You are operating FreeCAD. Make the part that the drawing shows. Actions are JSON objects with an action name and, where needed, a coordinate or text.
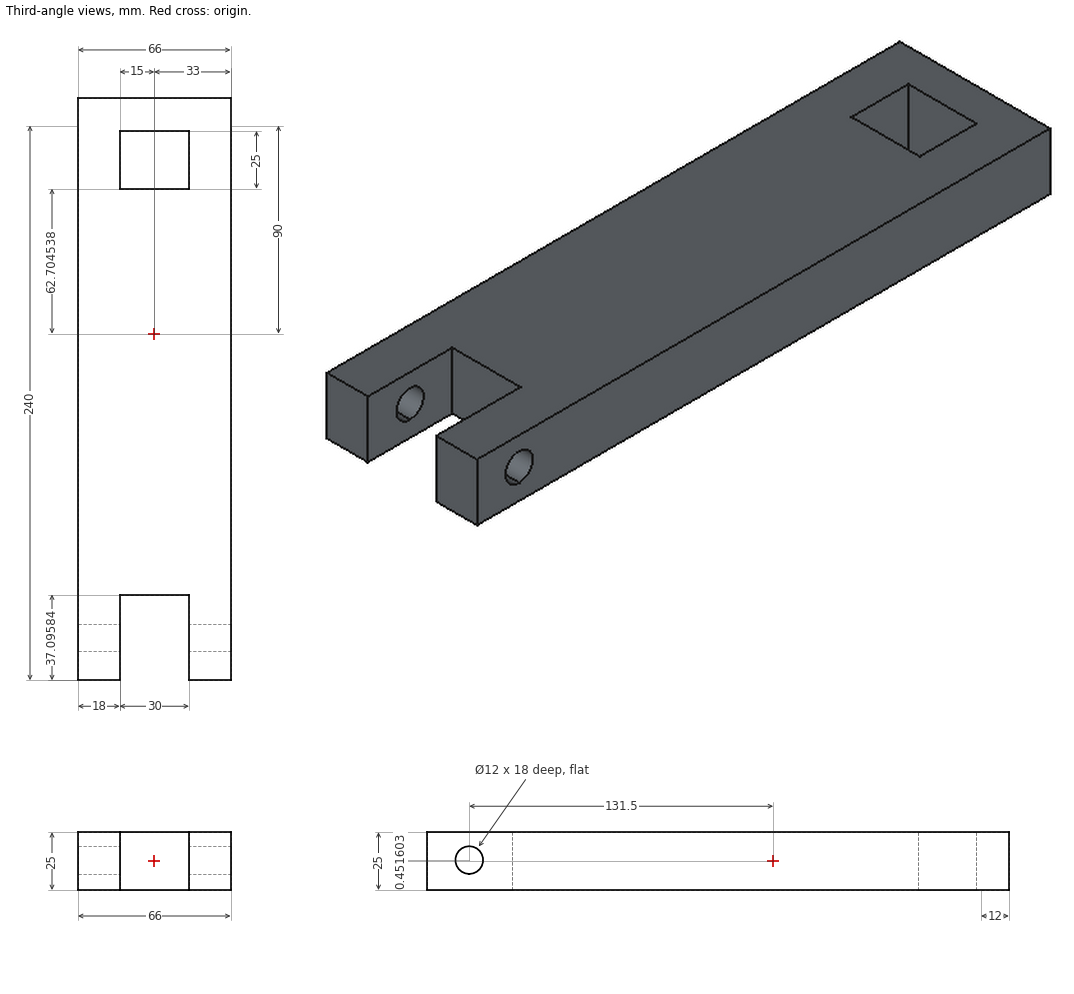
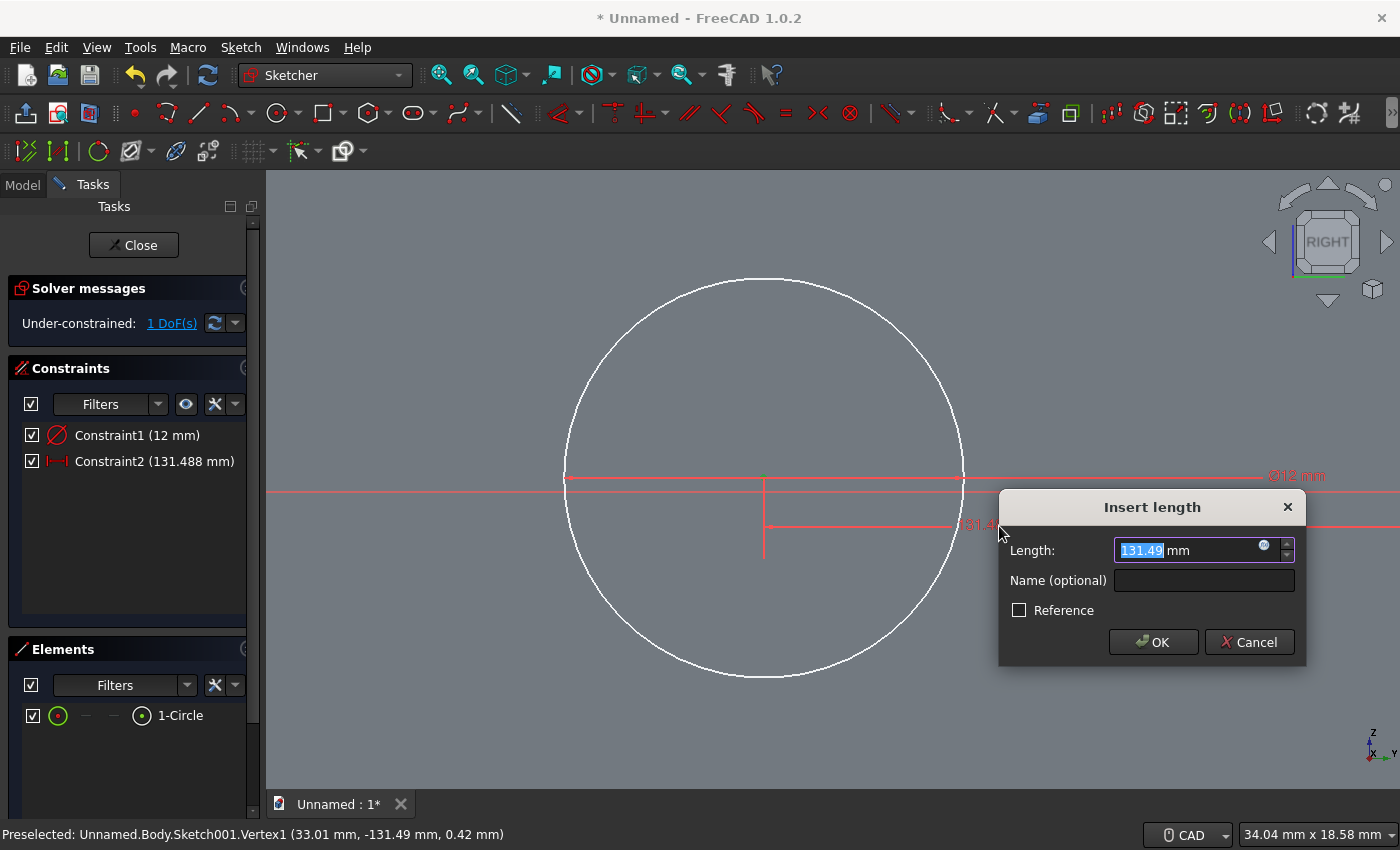
{"action": "type", "text": "131.5"}
{"action": "key", "text": "Return"}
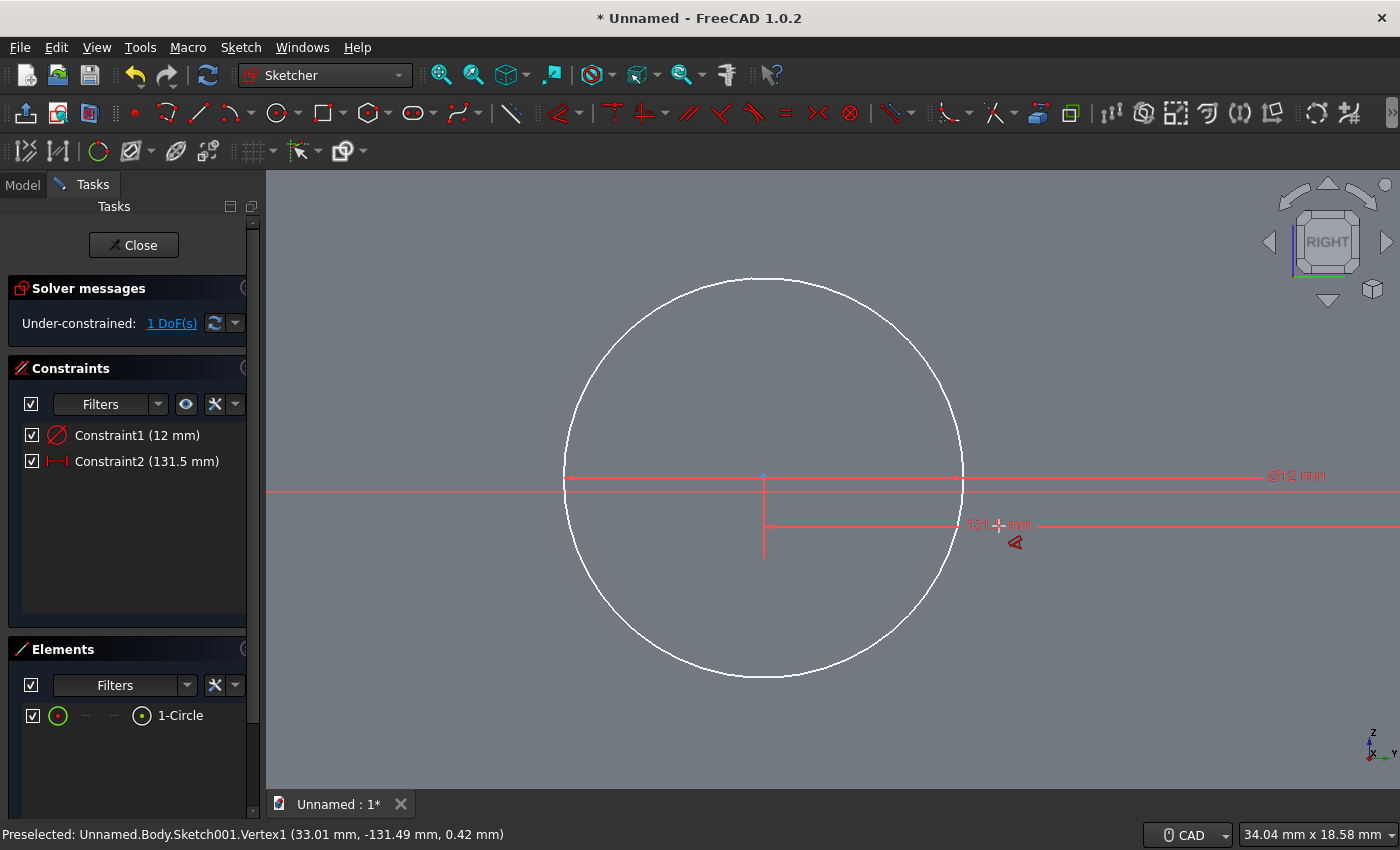
{"action": "scroll", "coordinate": [764, 478], "scroll_direction": "up", "scroll_amount": 5}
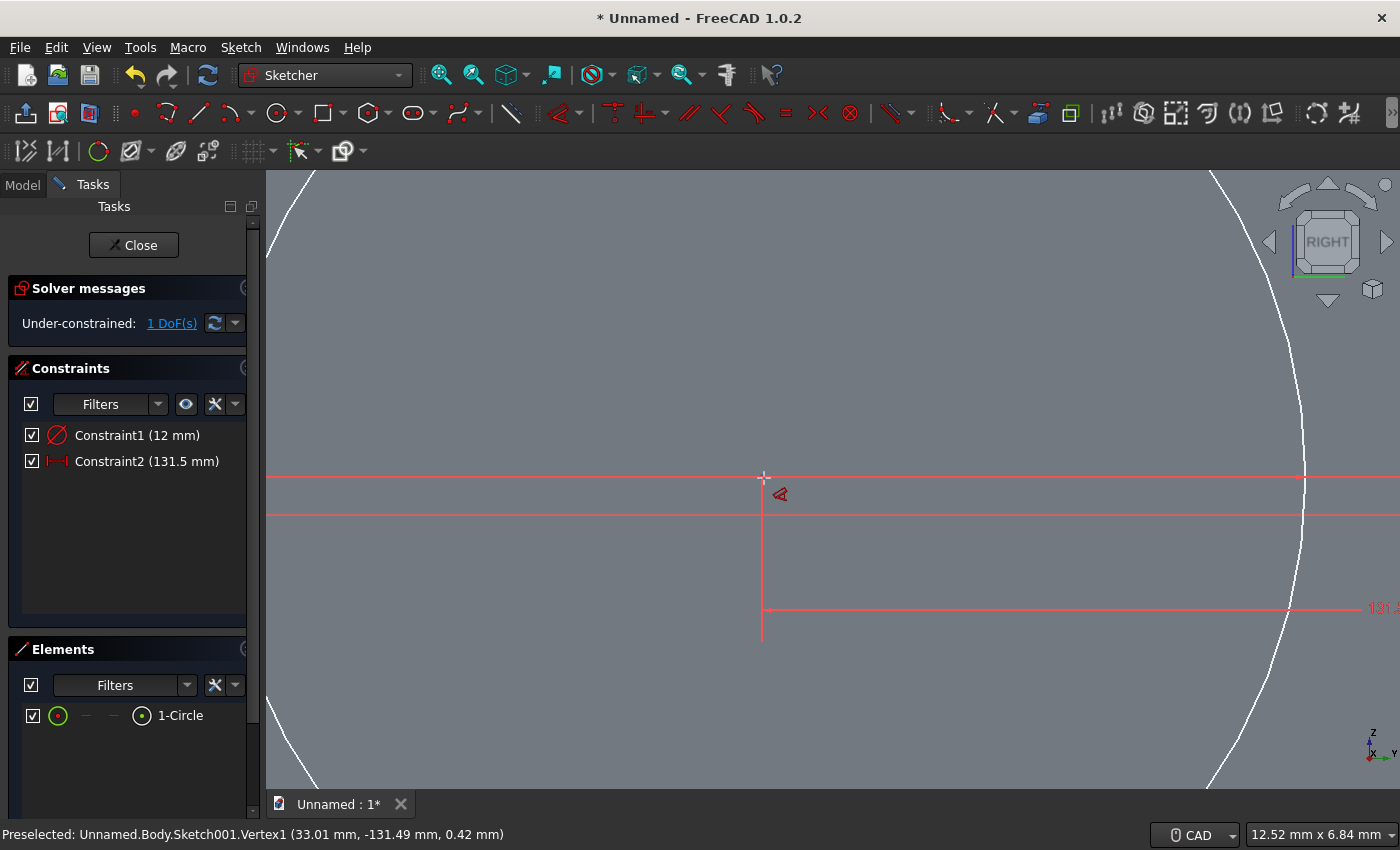
{"action": "left_click", "coordinate": [762, 477]}
{"action": "left_click", "coordinate": [728, 496]}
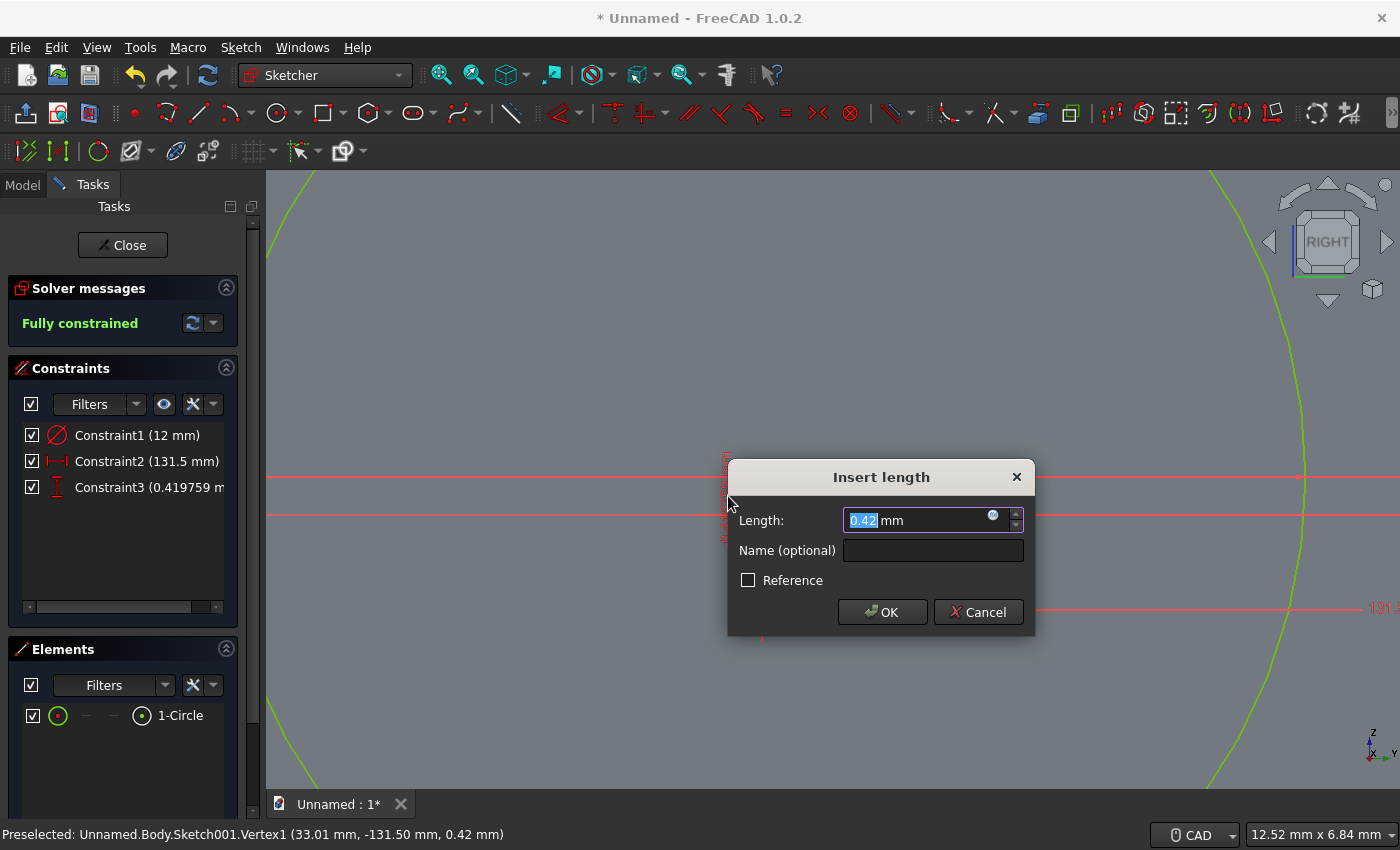
{"action": "type", "text": "0.451603"}
{"action": "key", "text": "Return"}
{"action": "key", "text": "Escape"}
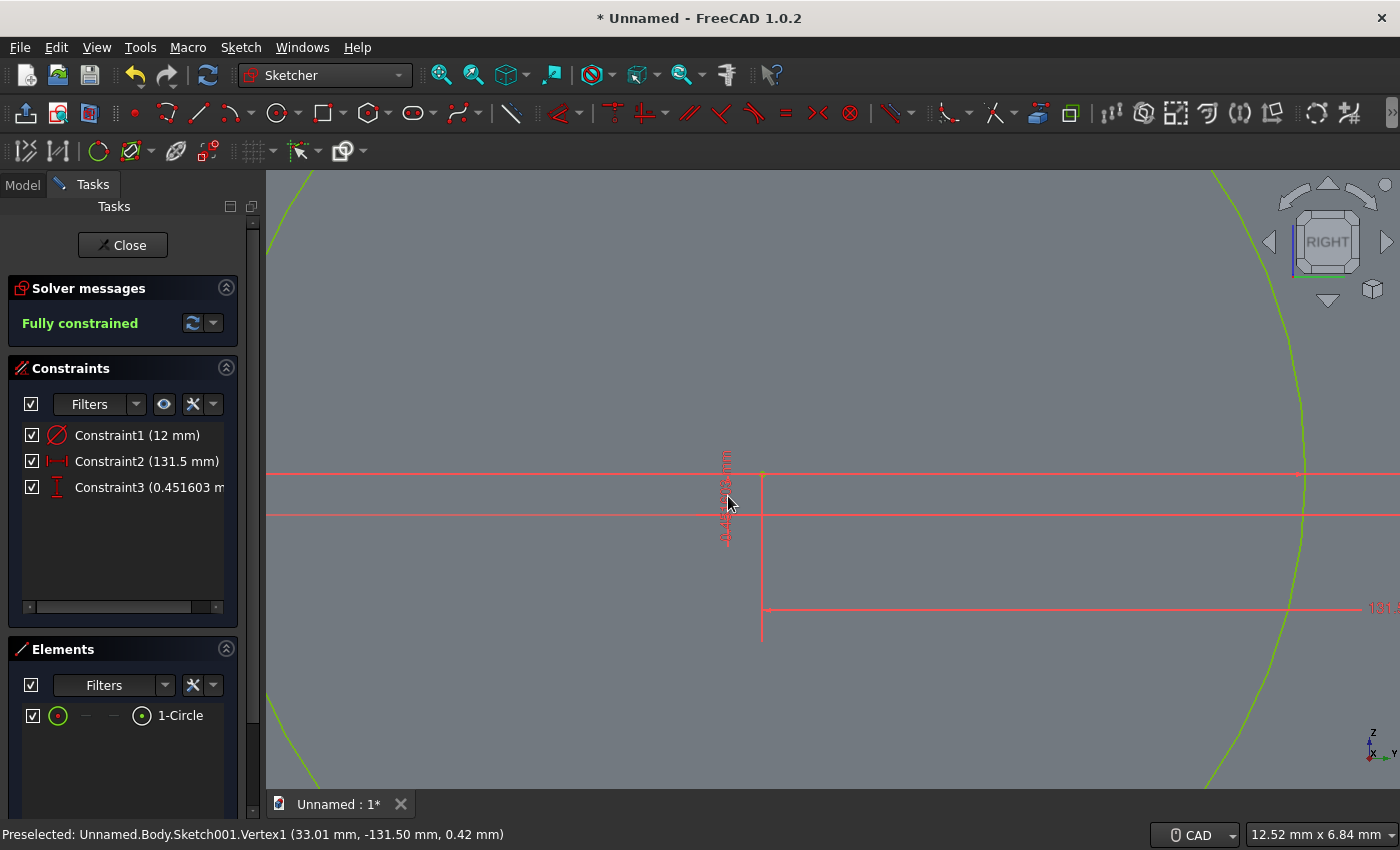
{"action": "left_click", "coordinate": [123, 245]}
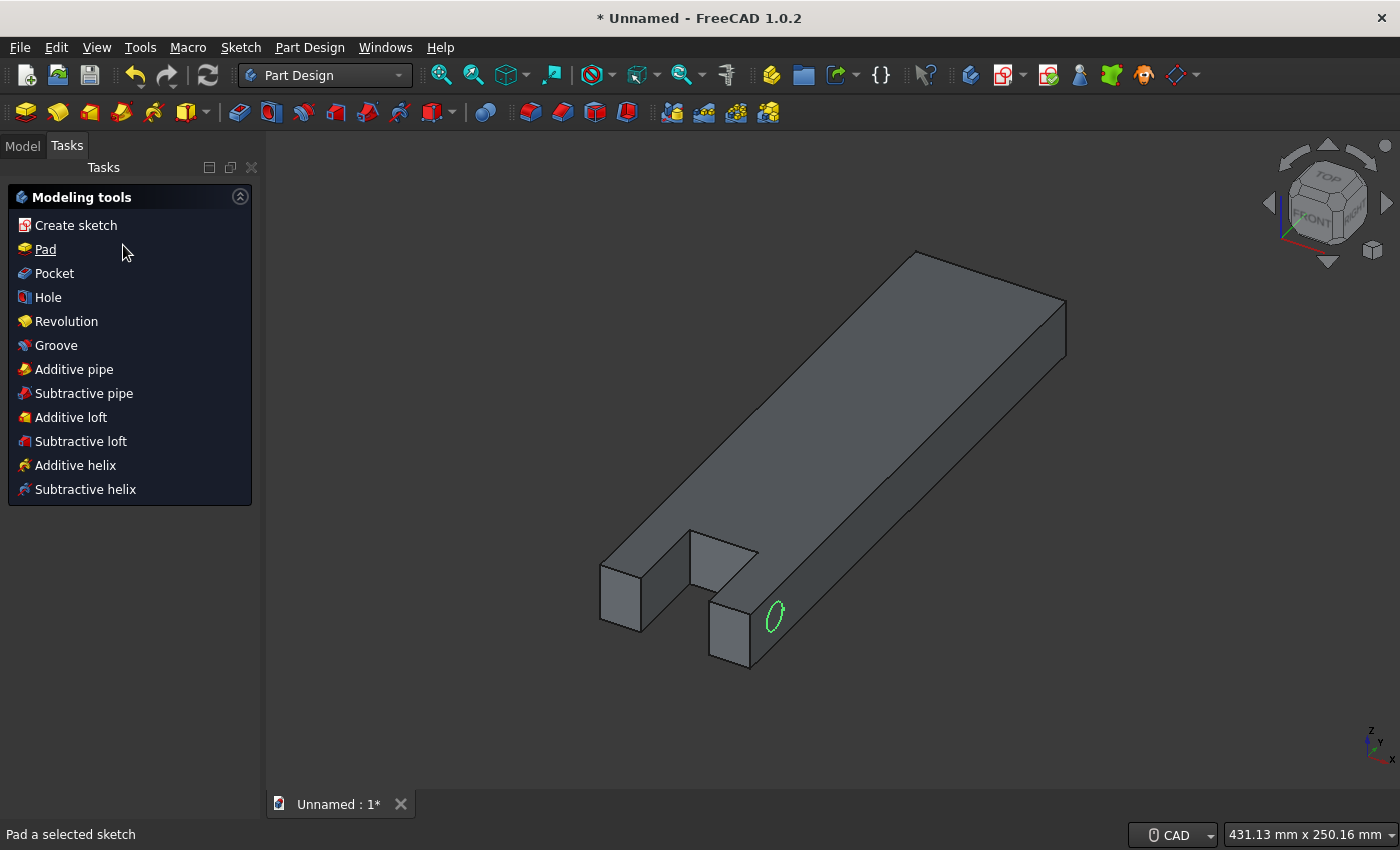
{"action": "left_click", "coordinate": [272, 112]}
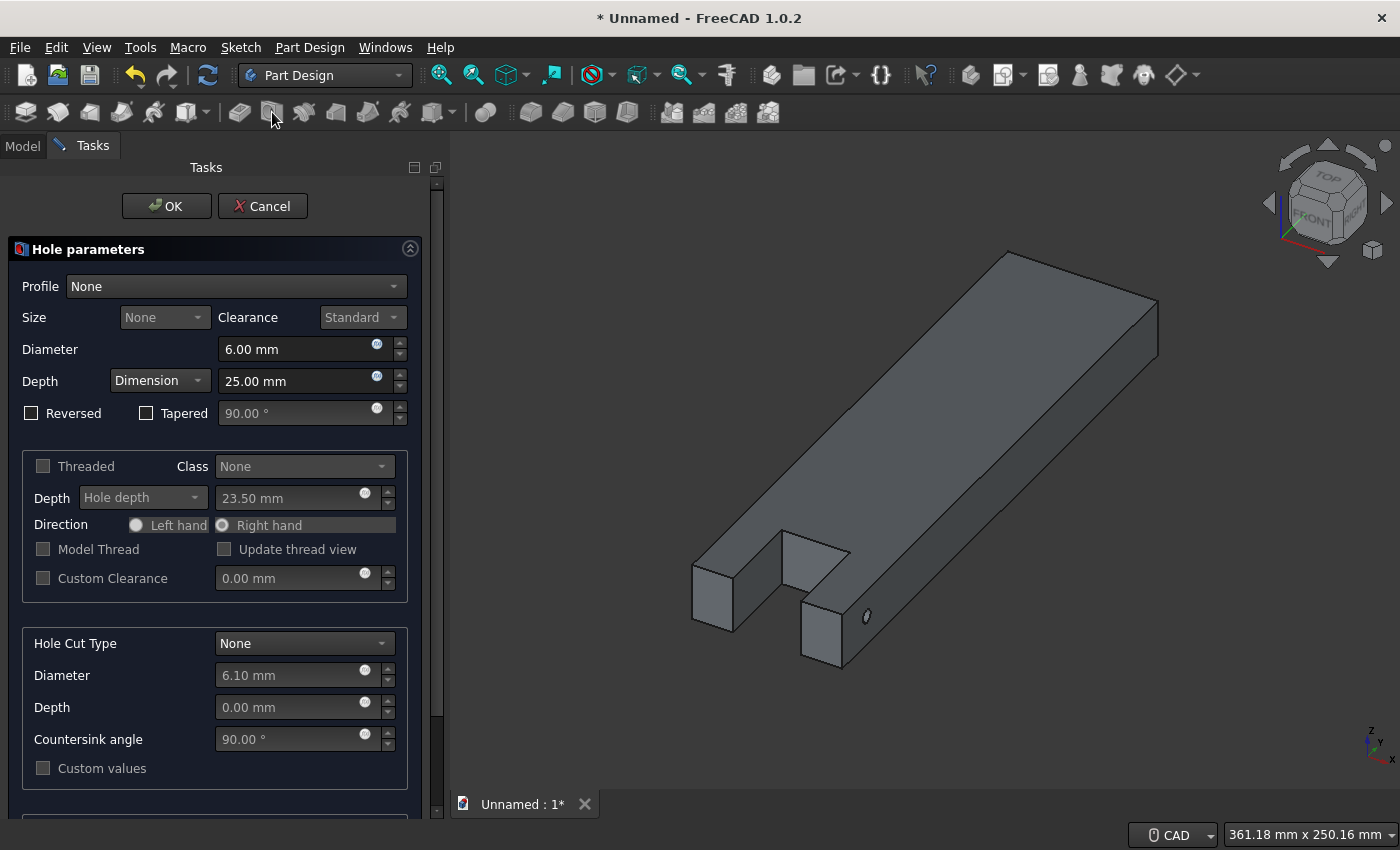
{"action": "triple_click", "coordinate": [305, 349]}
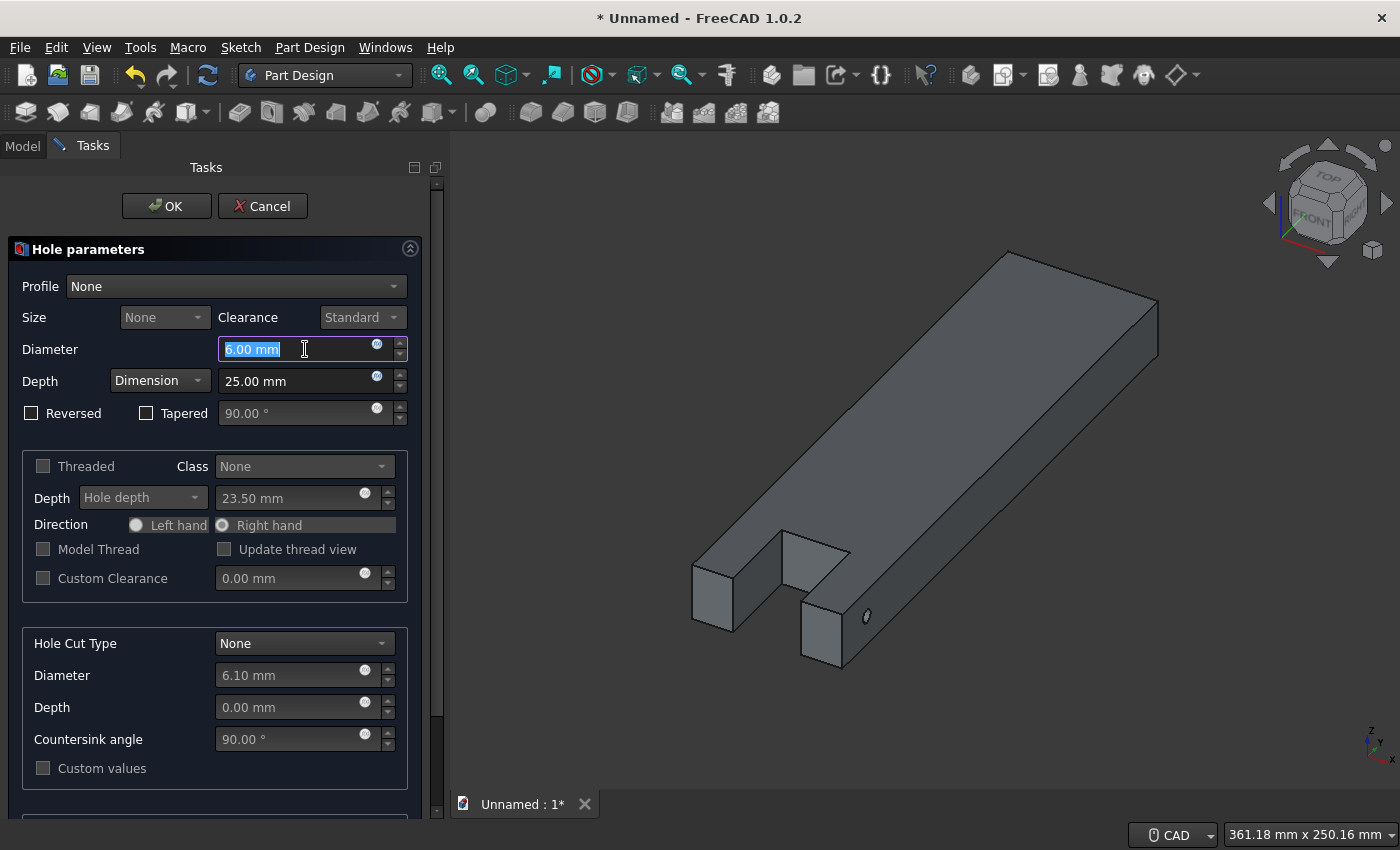
{"action": "type", "text": "12"}
{"action": "key", "text": "Tab"}